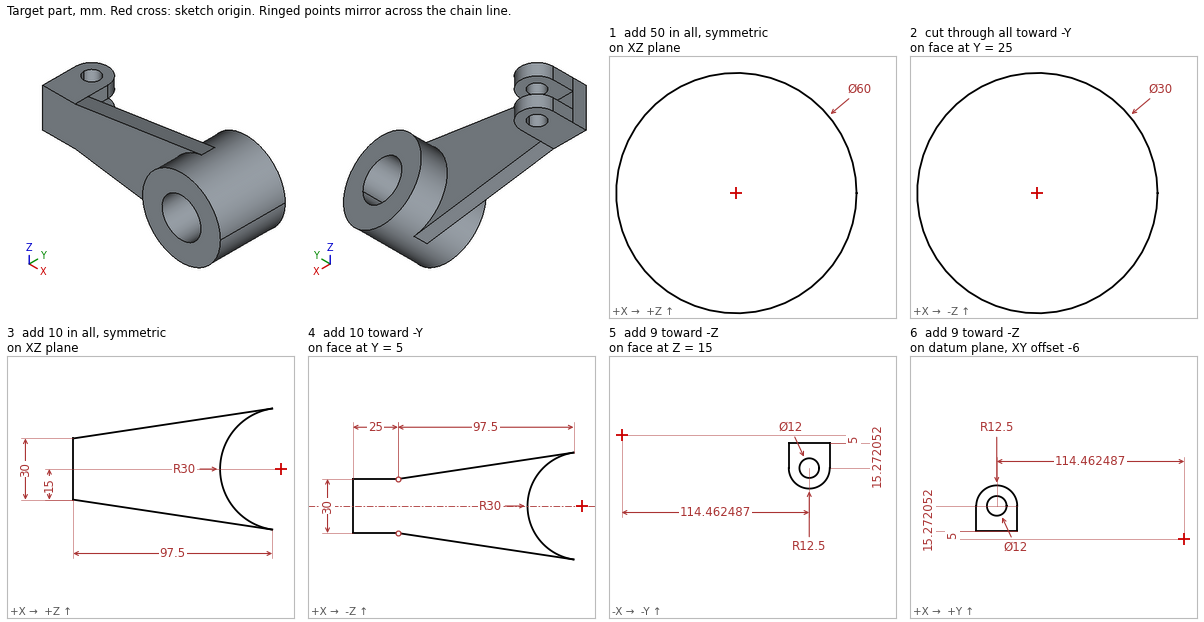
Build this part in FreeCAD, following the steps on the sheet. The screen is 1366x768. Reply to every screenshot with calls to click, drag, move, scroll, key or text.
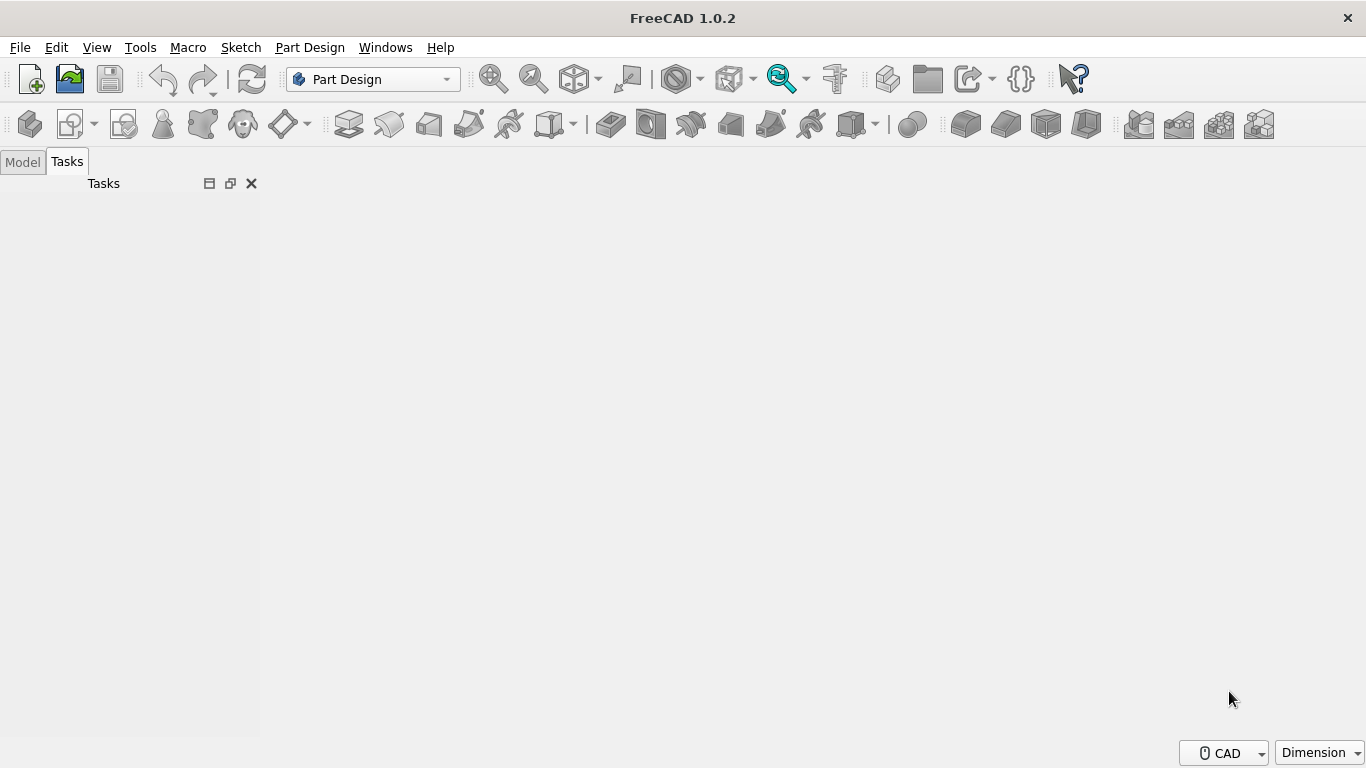
click(30, 80)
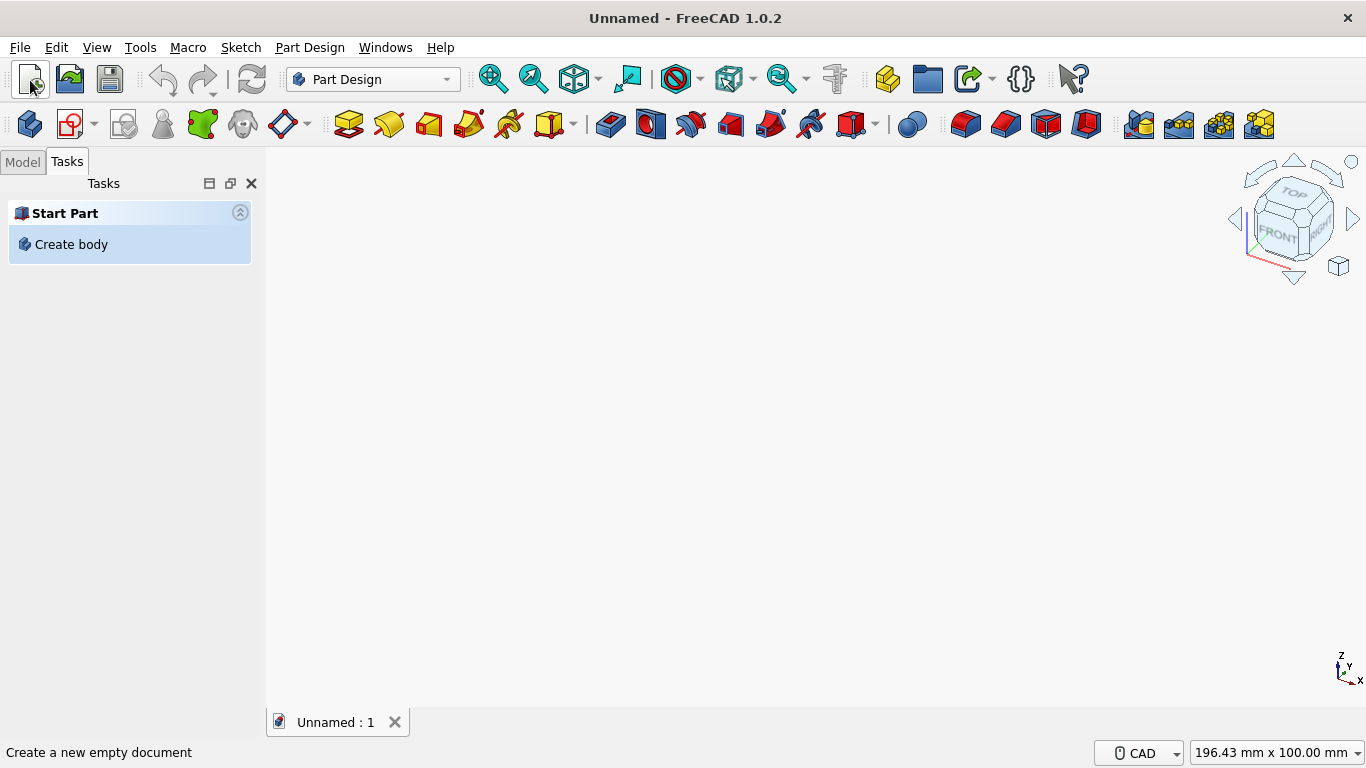
click(70, 124)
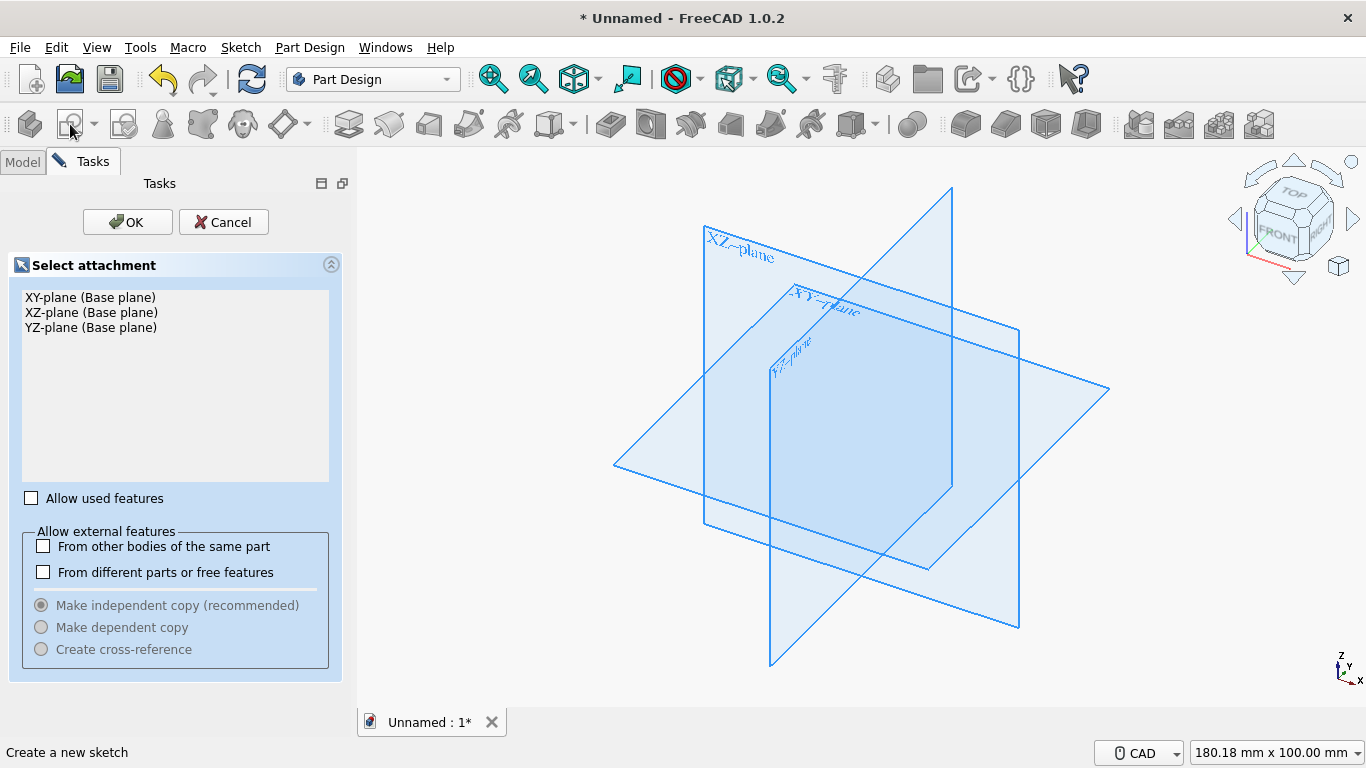
click(82, 312)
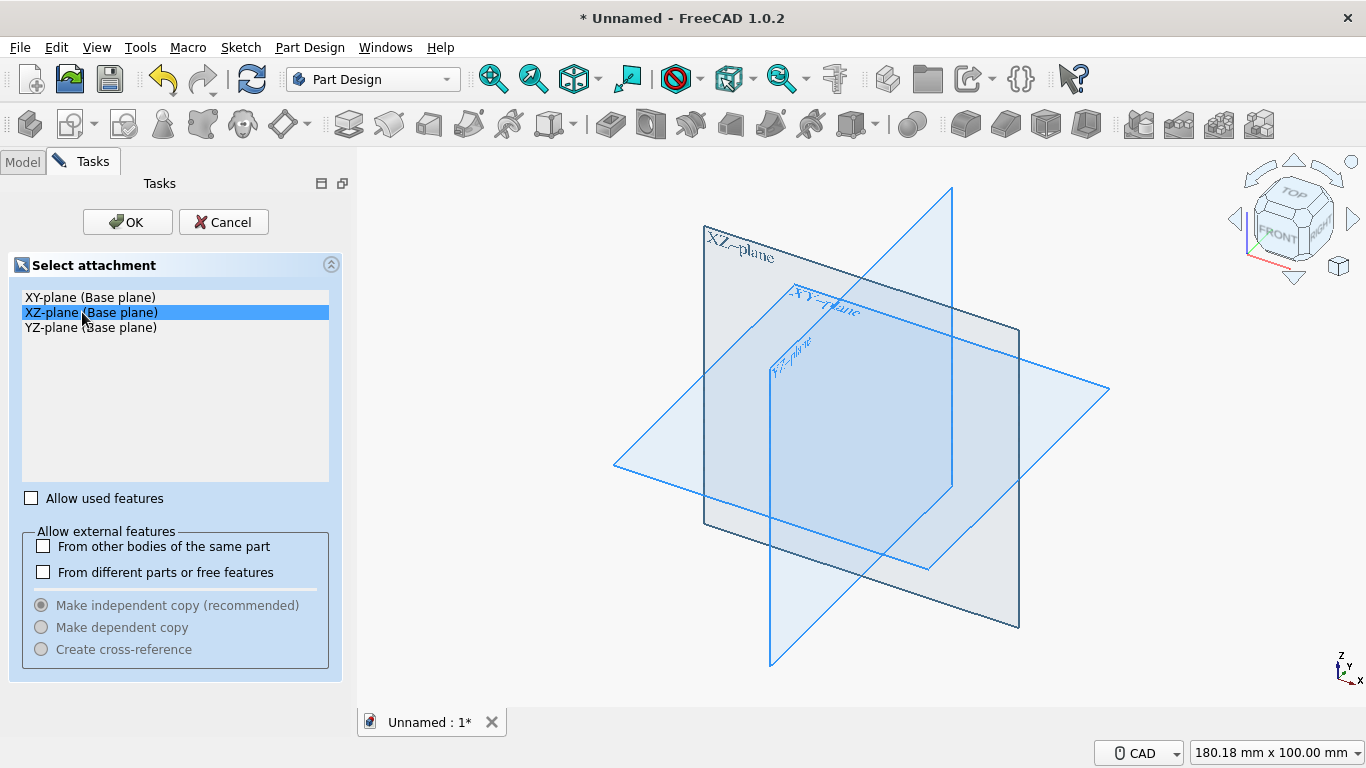
click(128, 222)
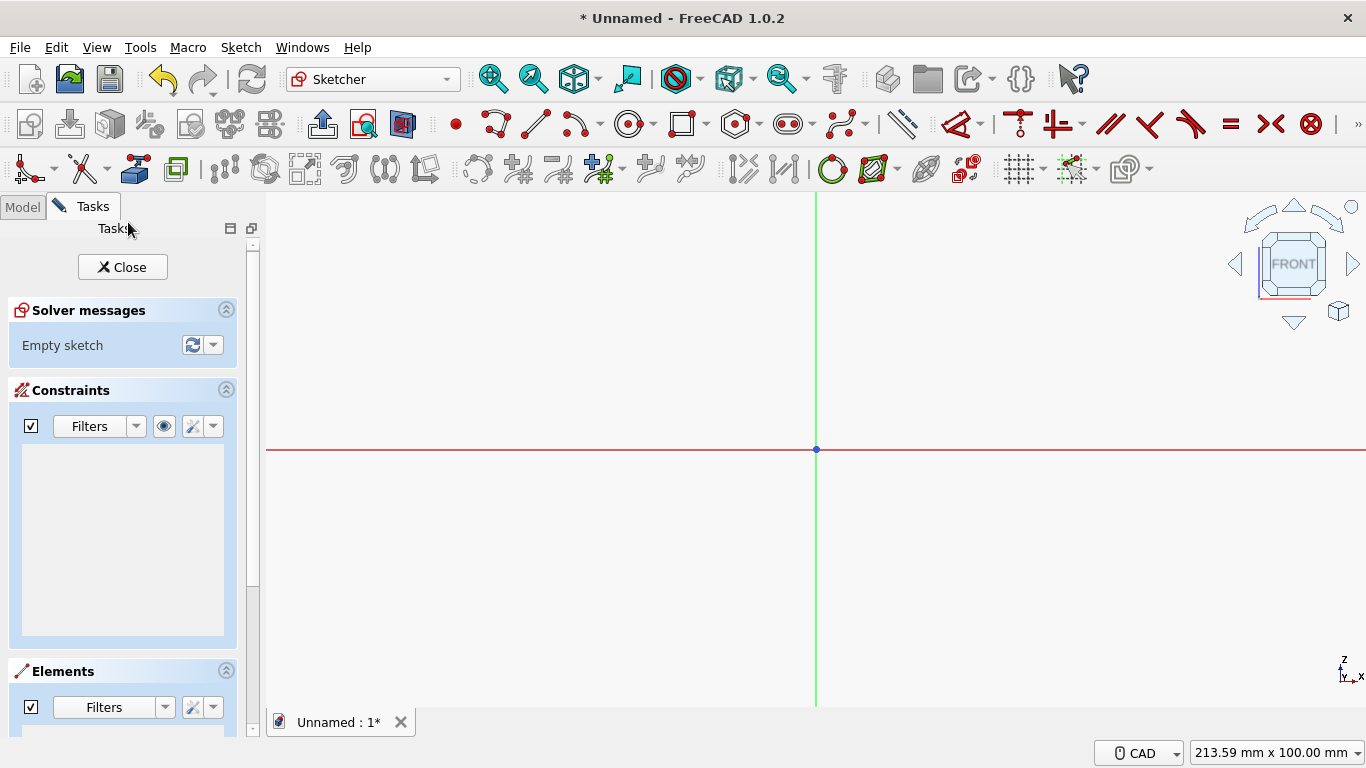
click(630, 124)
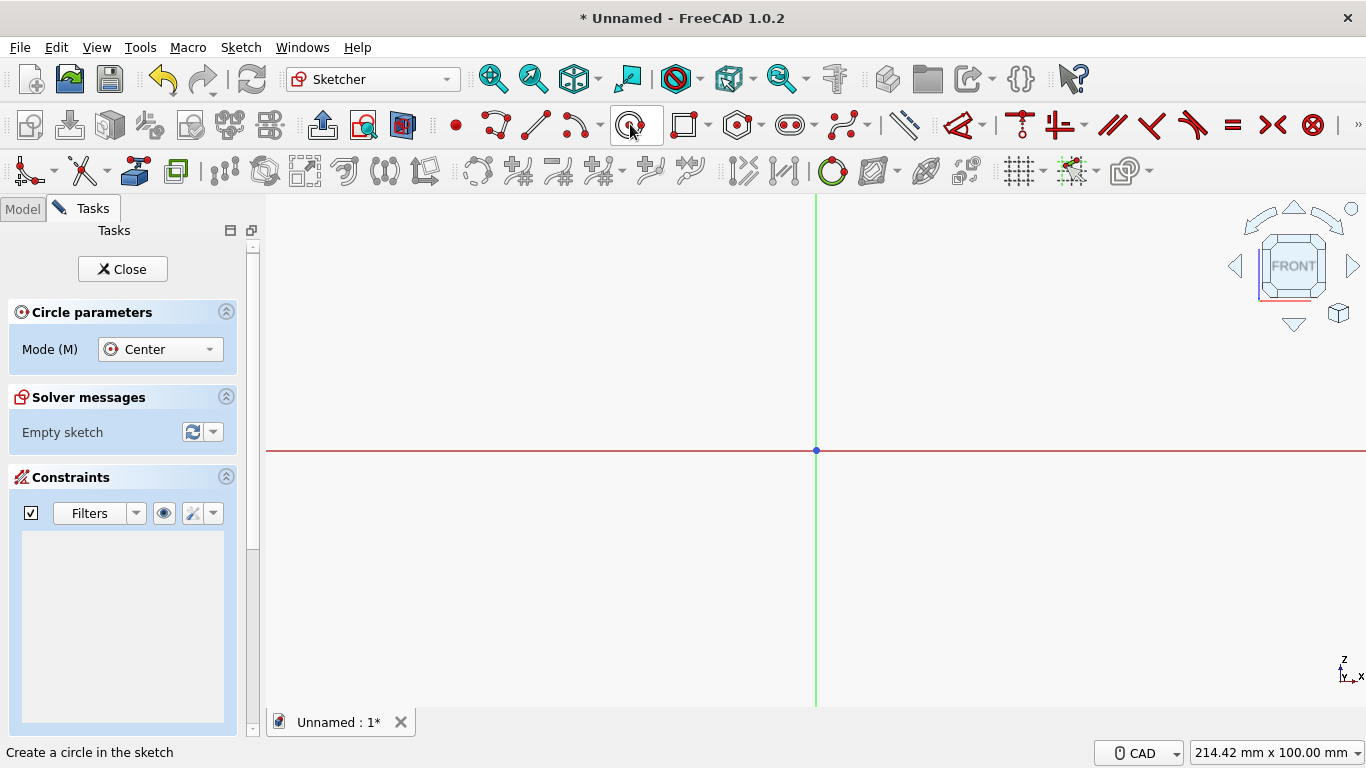
click(816, 450)
move(925, 342)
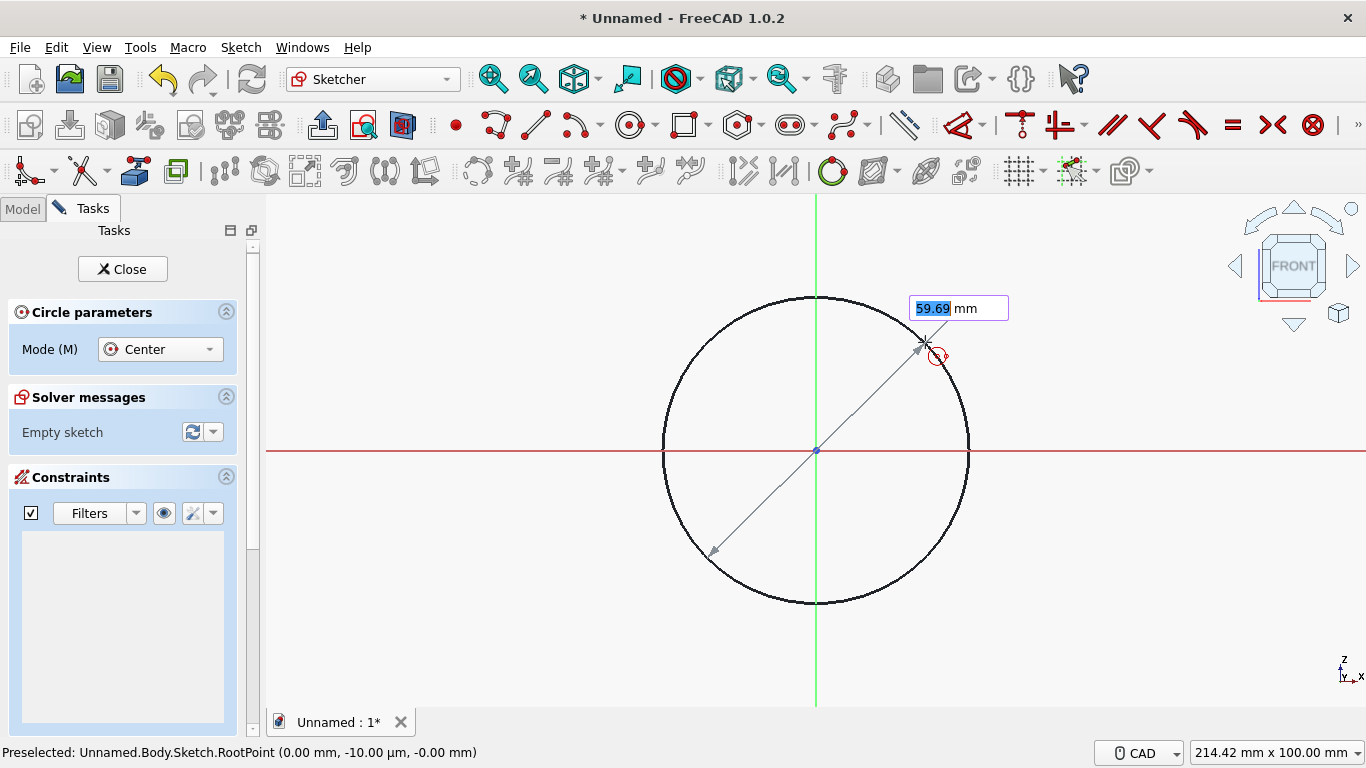
text(60)
key(Return)
key(Escape)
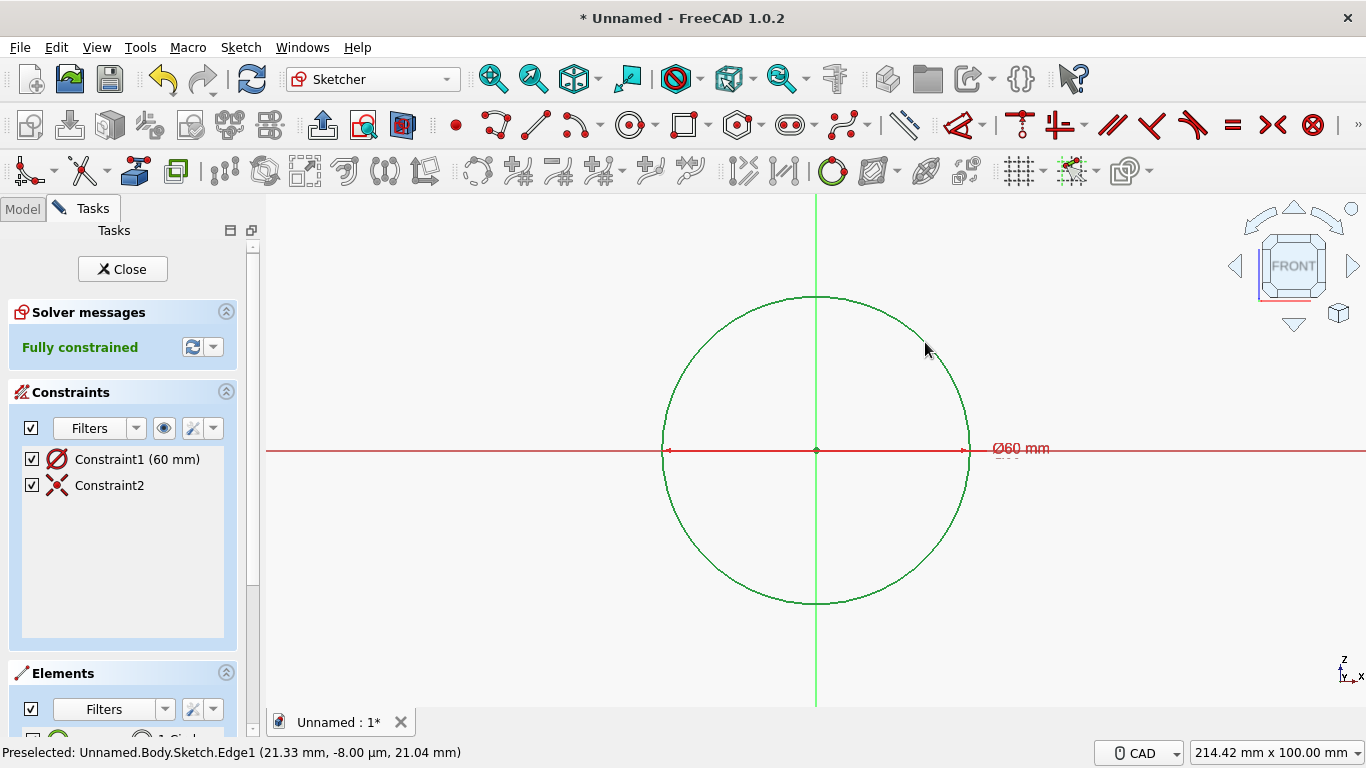
click(123, 269)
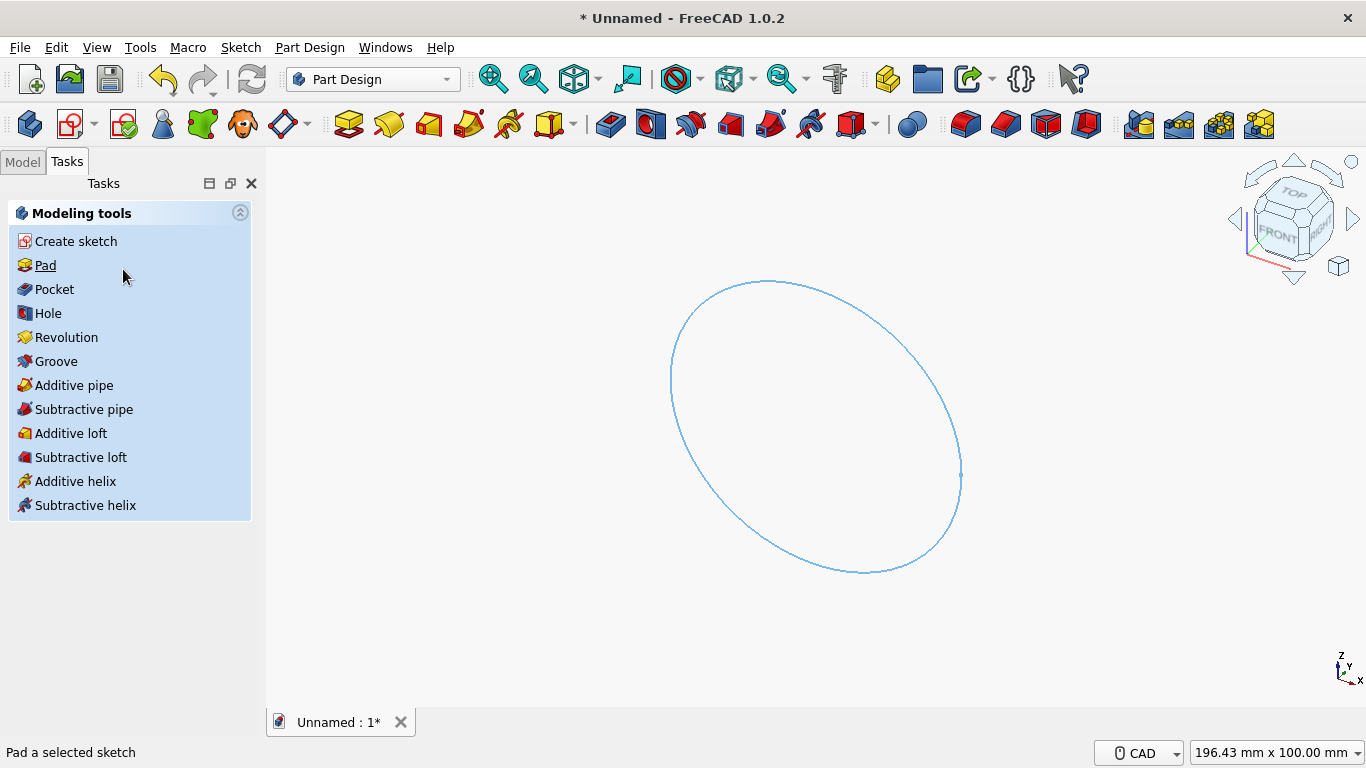
click(350, 124)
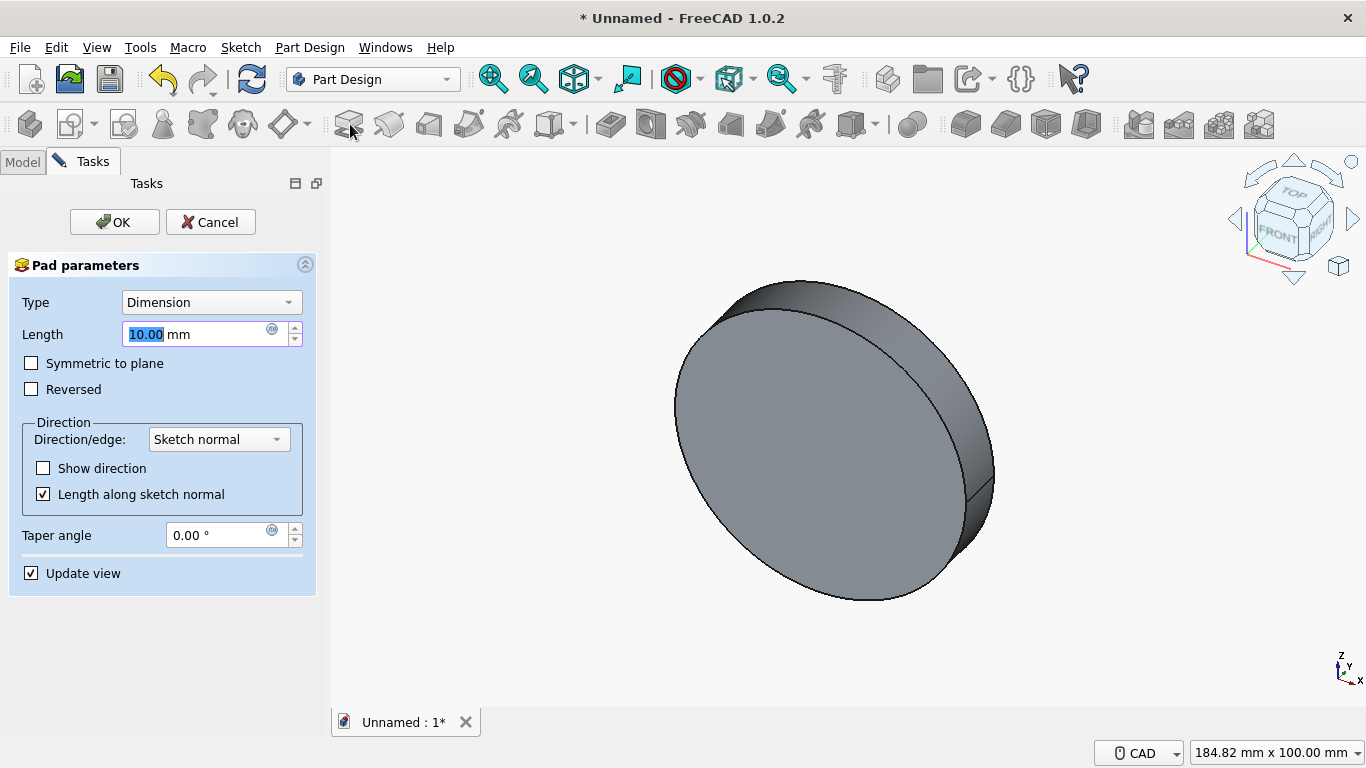
text(50)
key(Tab)